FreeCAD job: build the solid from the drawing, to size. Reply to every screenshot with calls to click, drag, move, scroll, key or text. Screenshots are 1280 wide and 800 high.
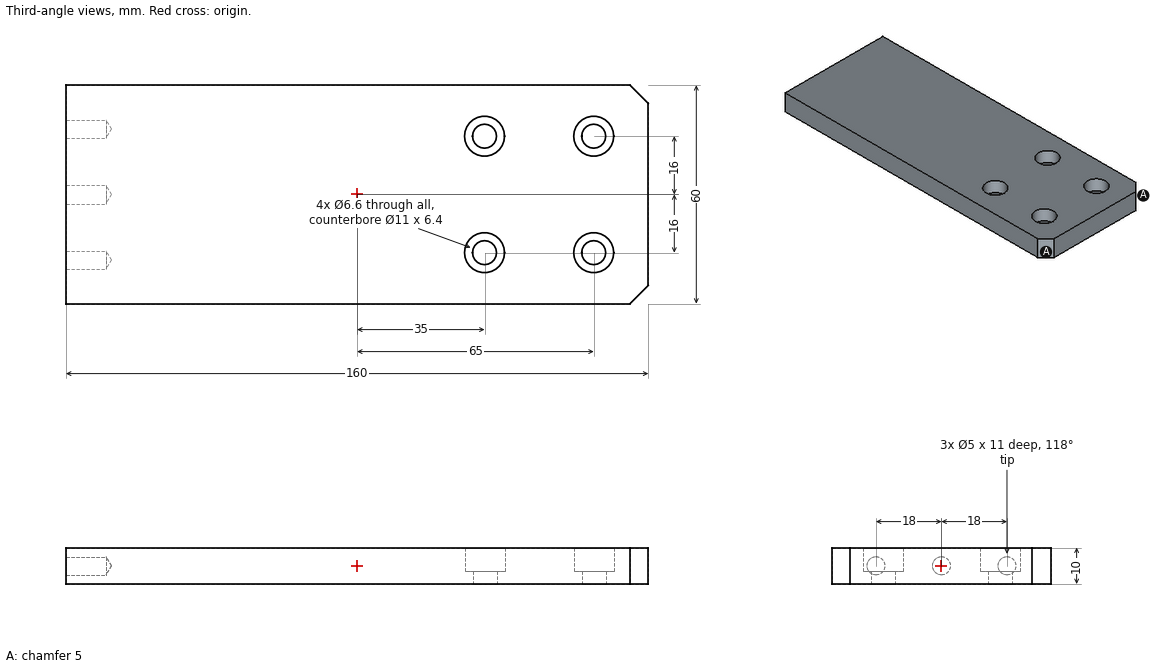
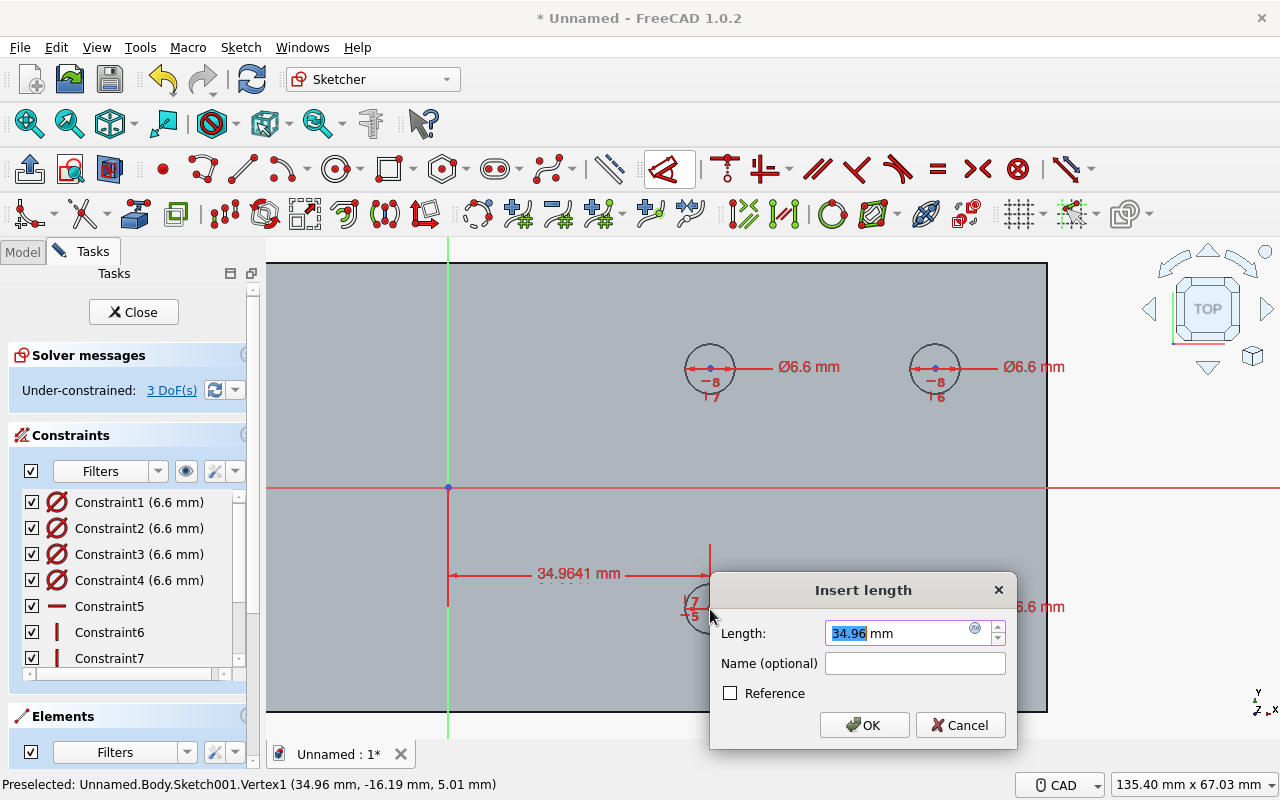
text(35)
key(Return)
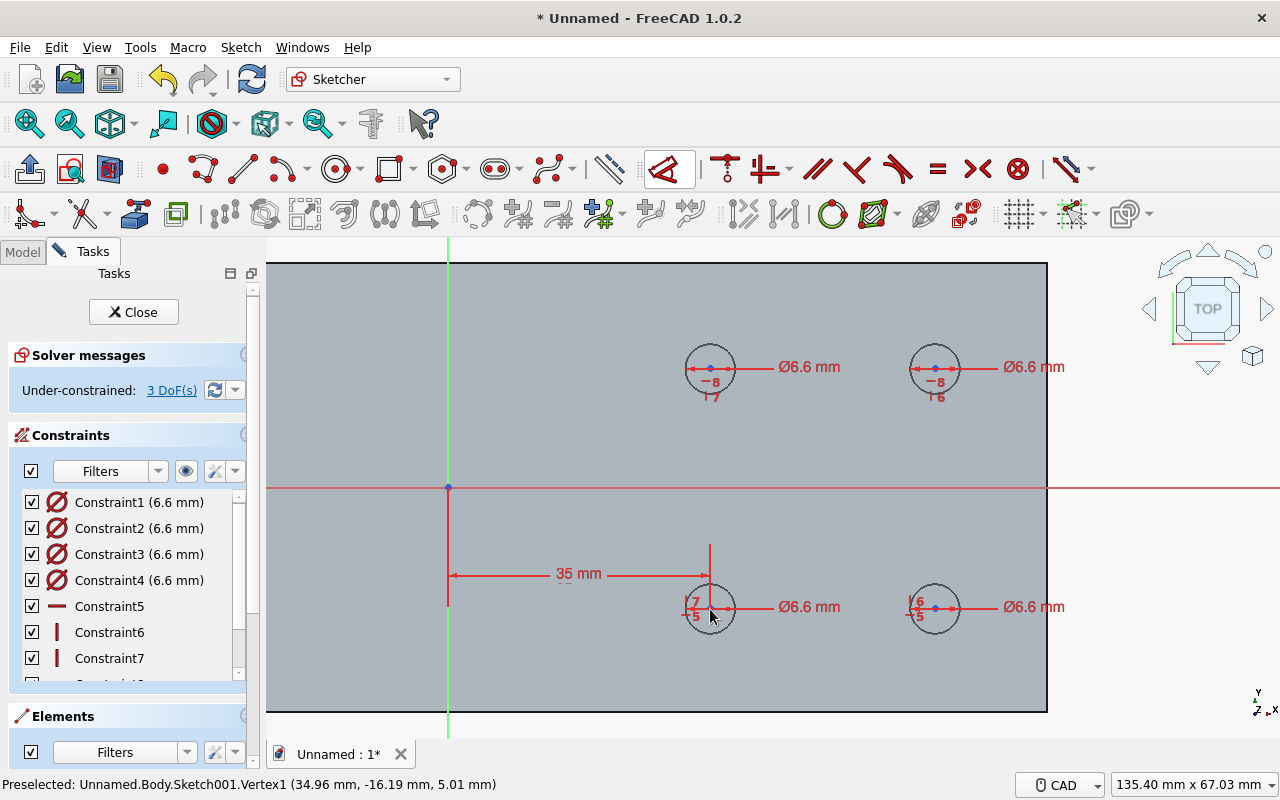
click(710, 609)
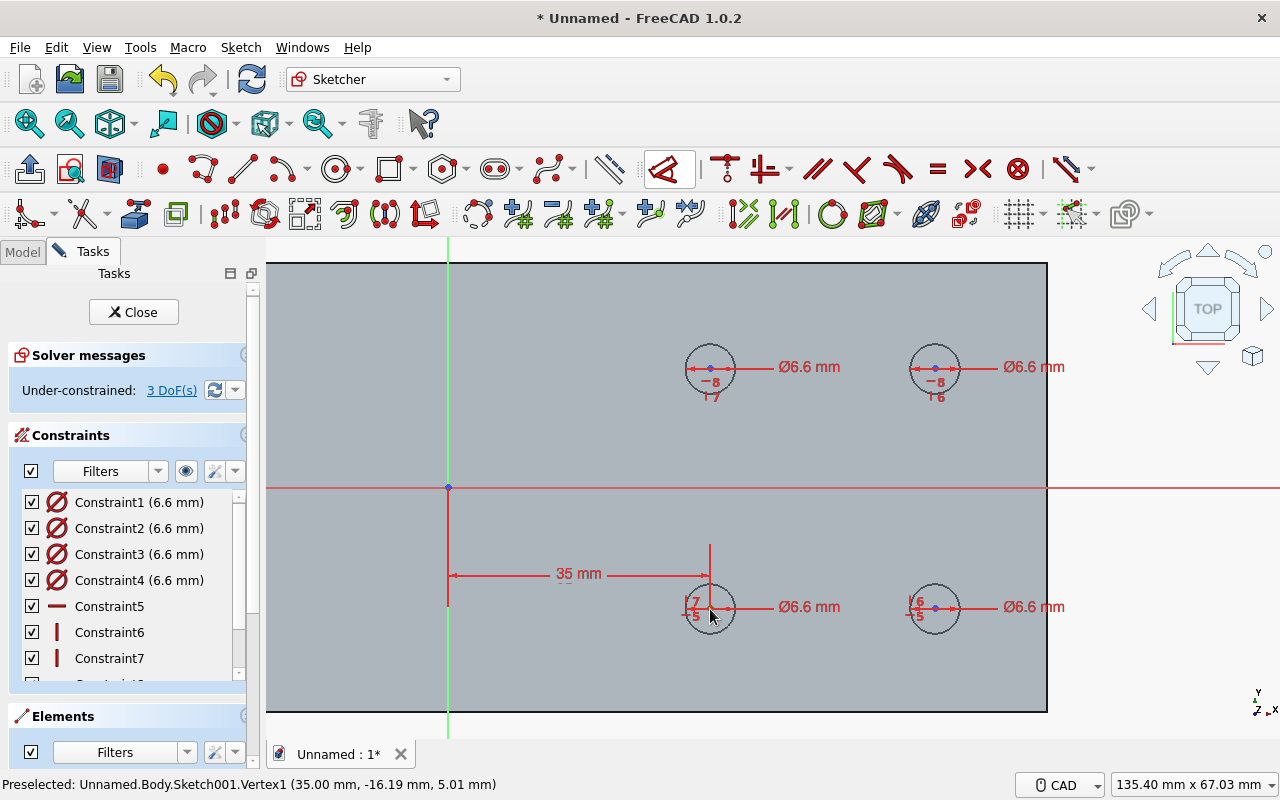
key(i)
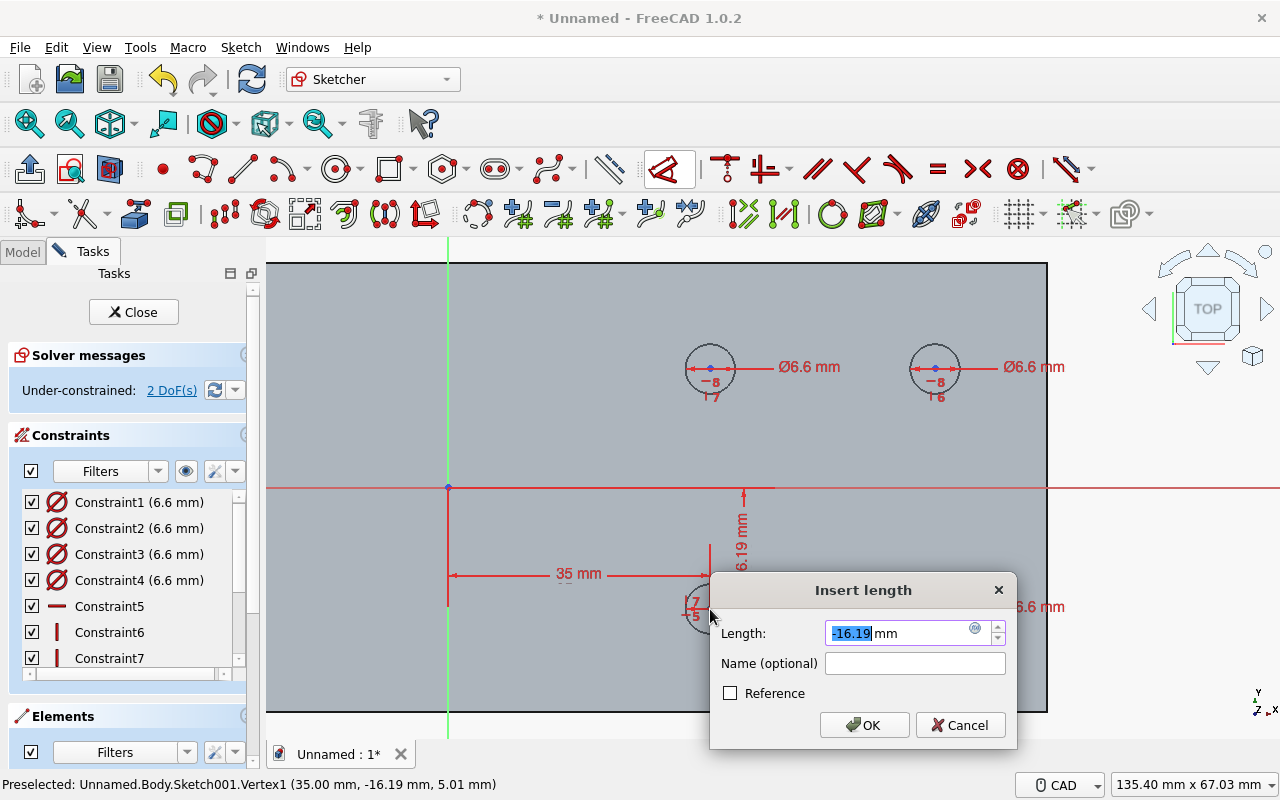
text(-16)
key(Return)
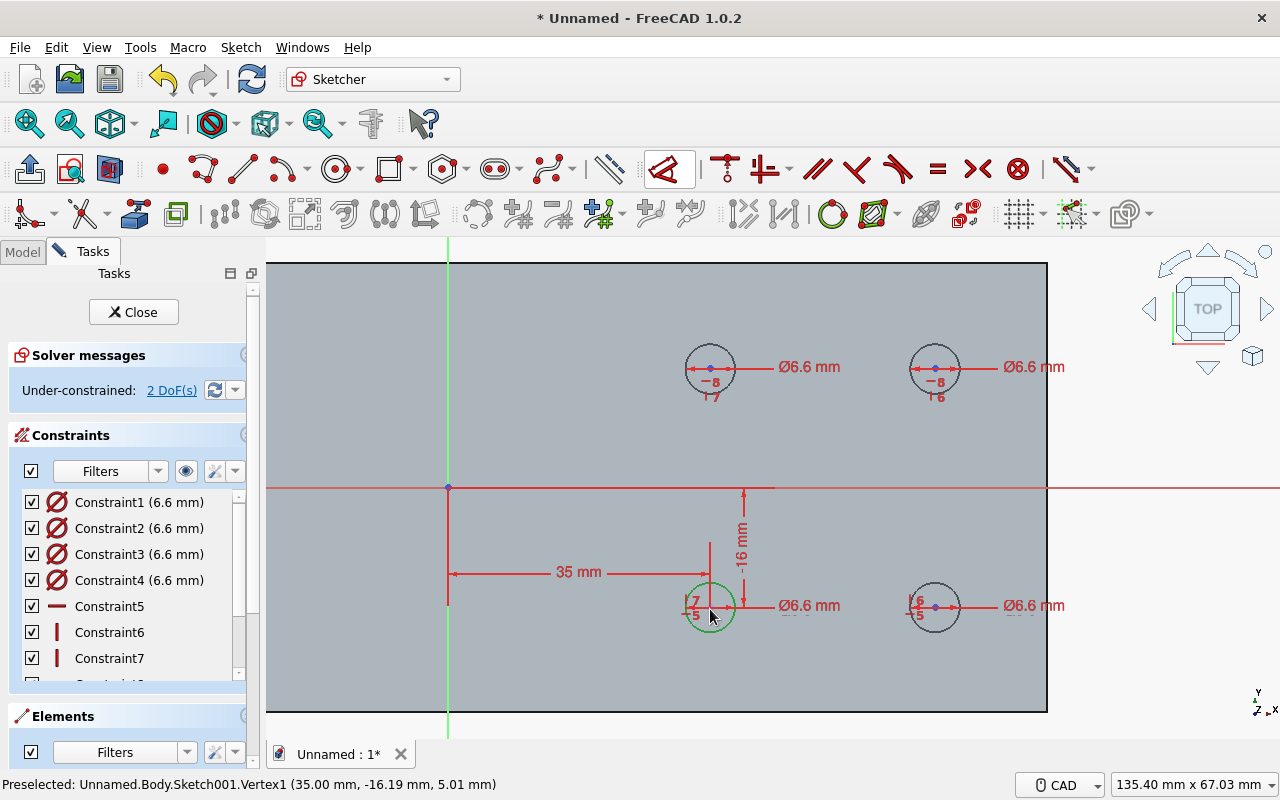
click(935, 608)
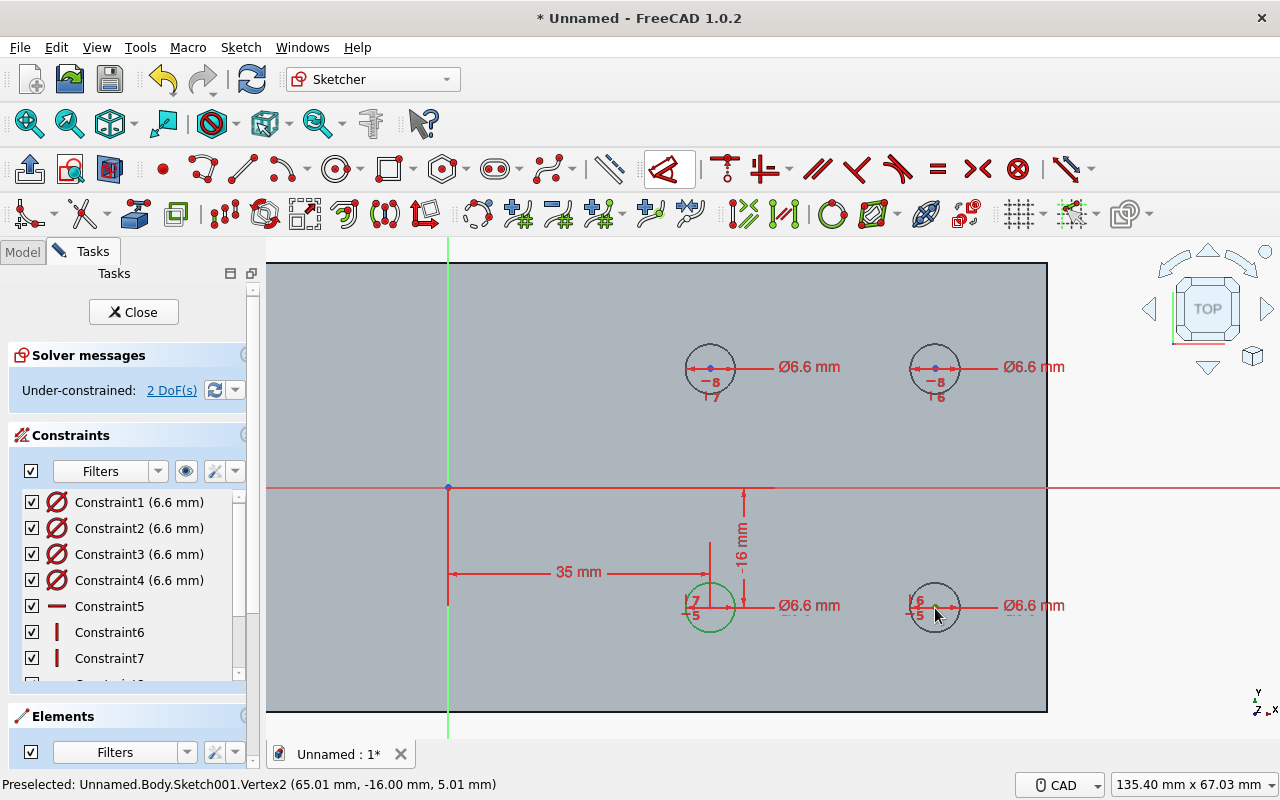
key(l)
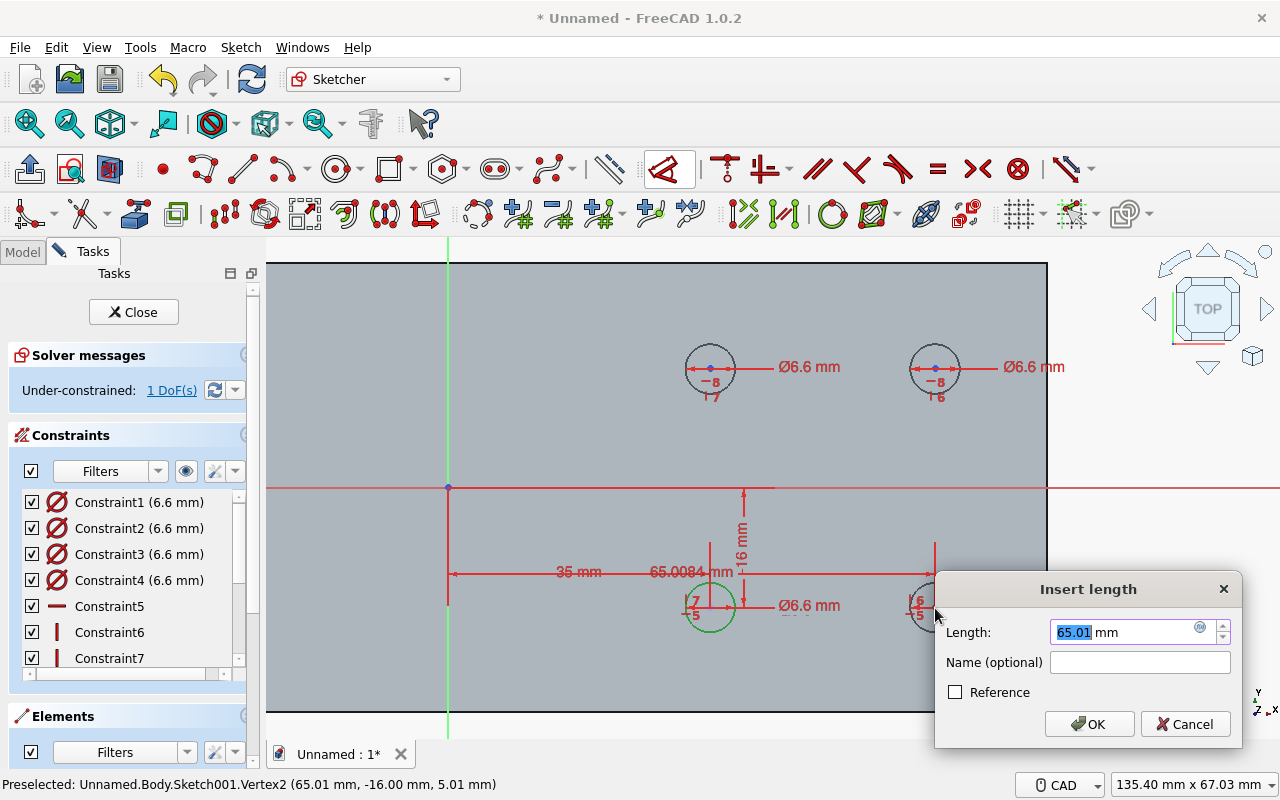
text(65)
key(Return)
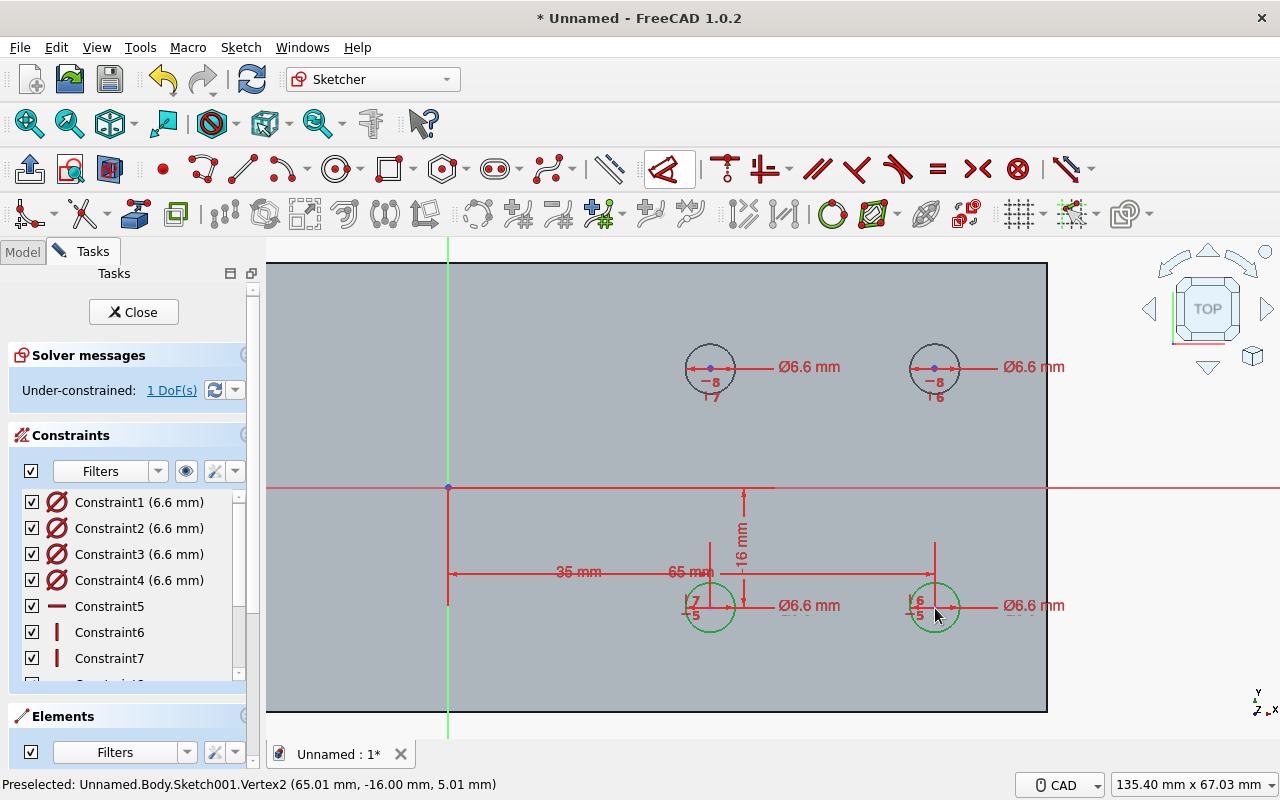
click(935, 369)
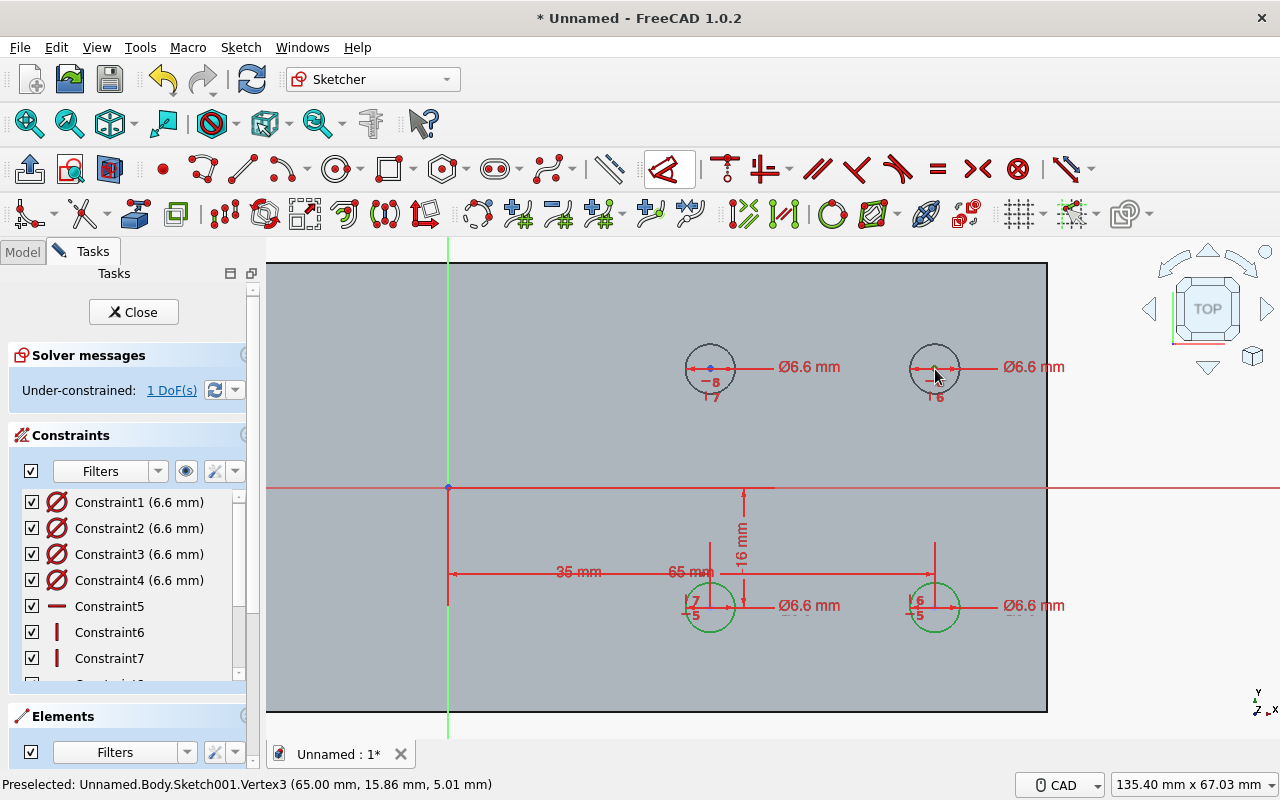
key(i)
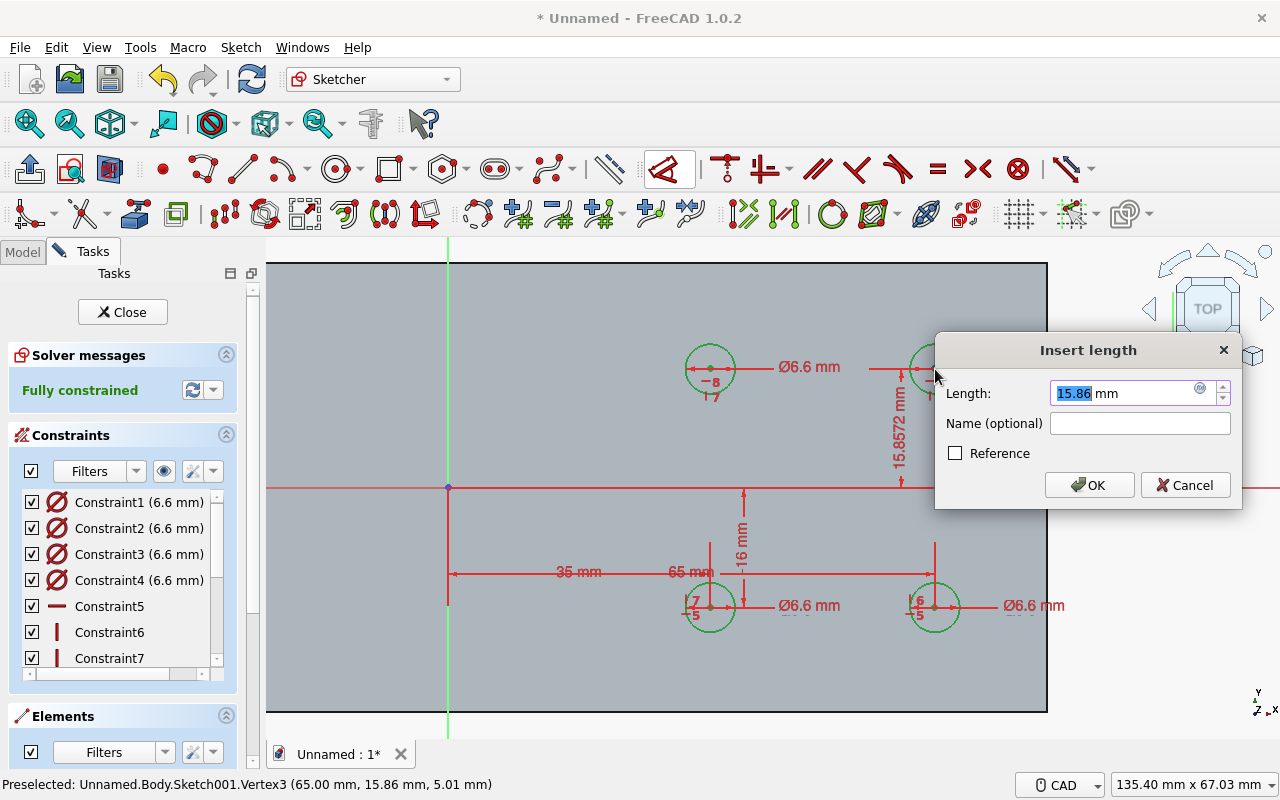
text(16)
key(Return)